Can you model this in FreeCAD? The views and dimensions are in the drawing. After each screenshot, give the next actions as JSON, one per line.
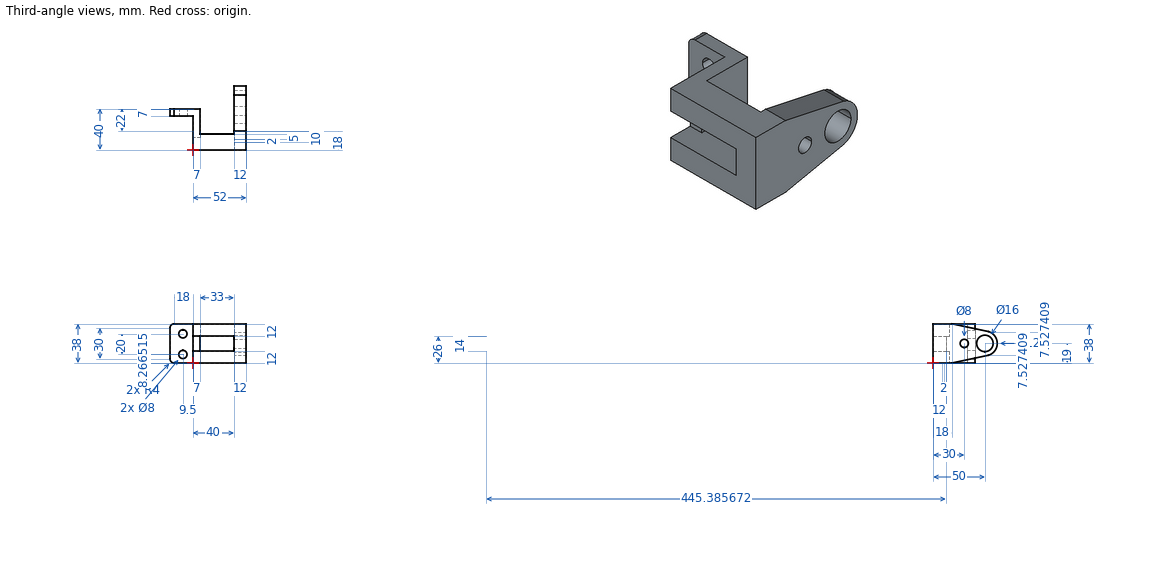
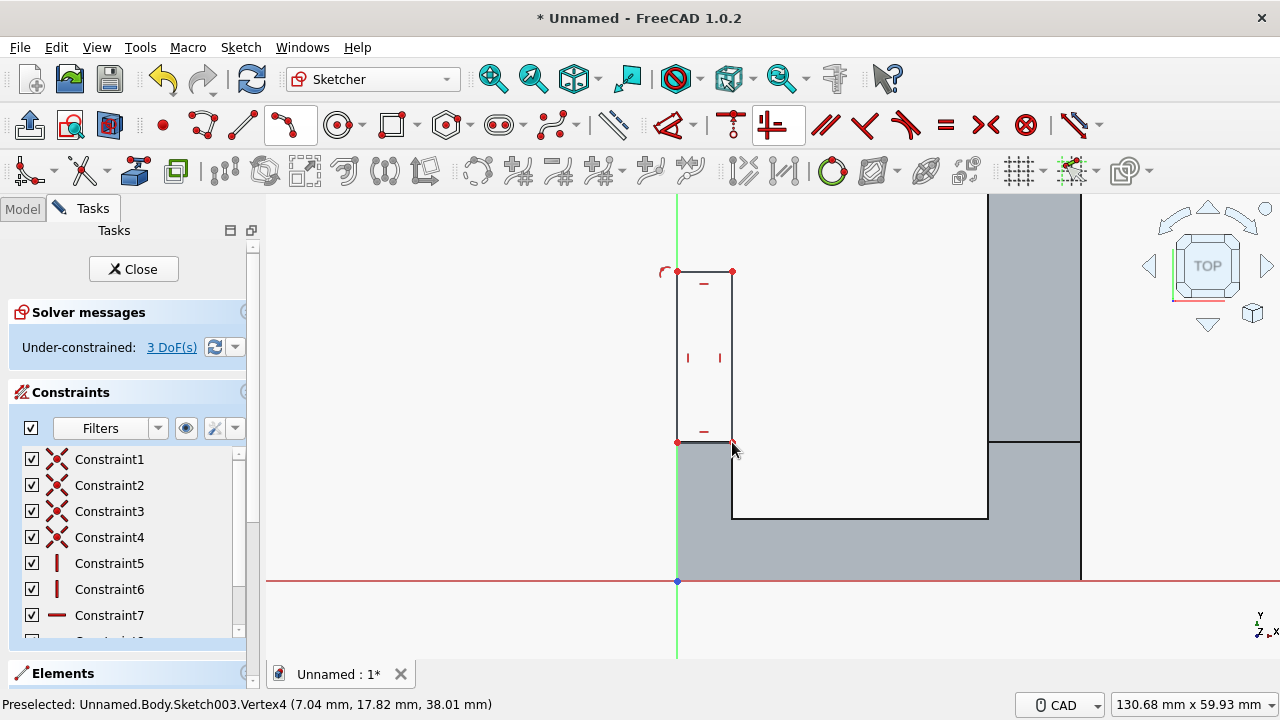
{"action": "left_click", "coordinate": [668, 126]}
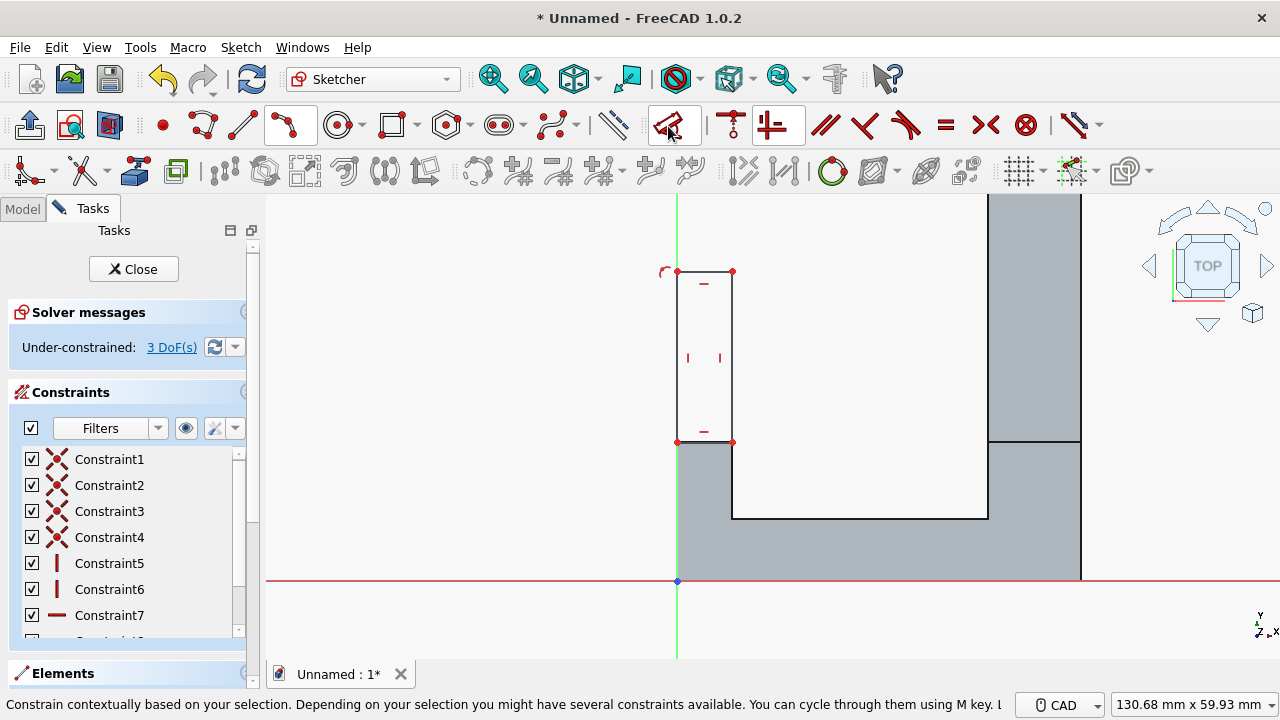
{"action": "left_click", "coordinate": [694, 443]}
{"action": "left_click", "coordinate": [705, 477]}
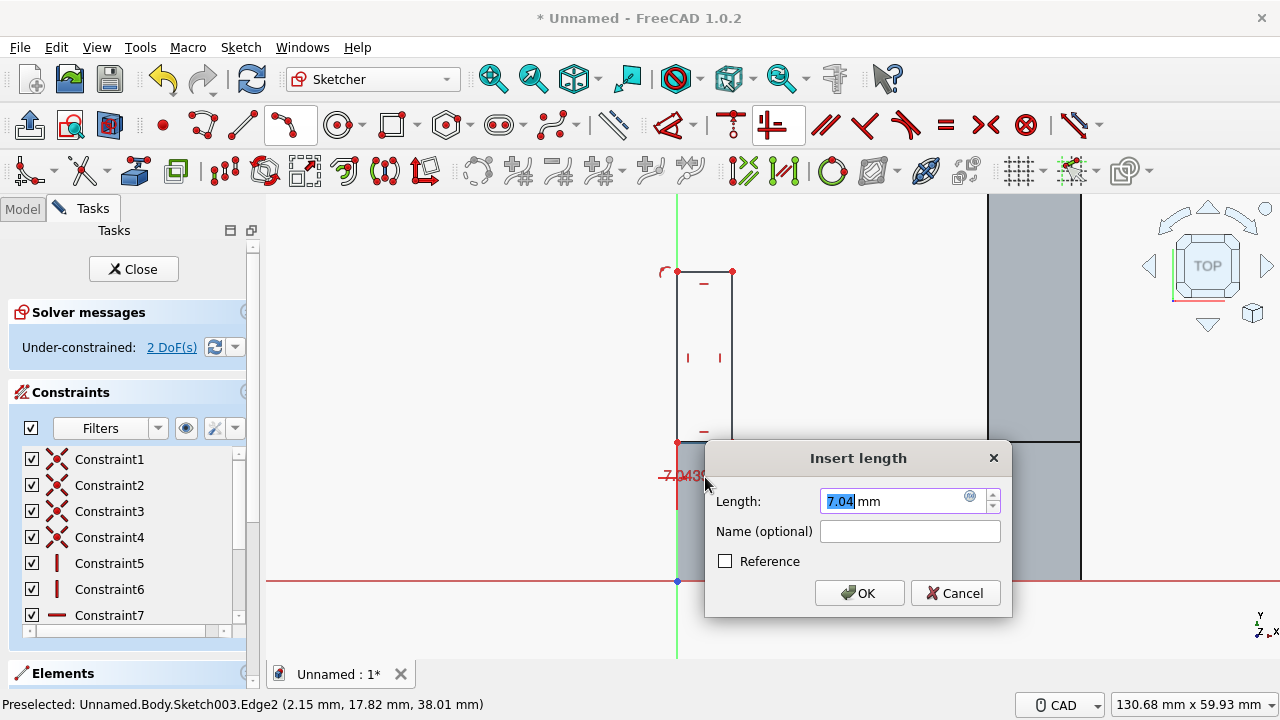
{"action": "type", "text": "7"}
{"action": "key", "text": "Return"}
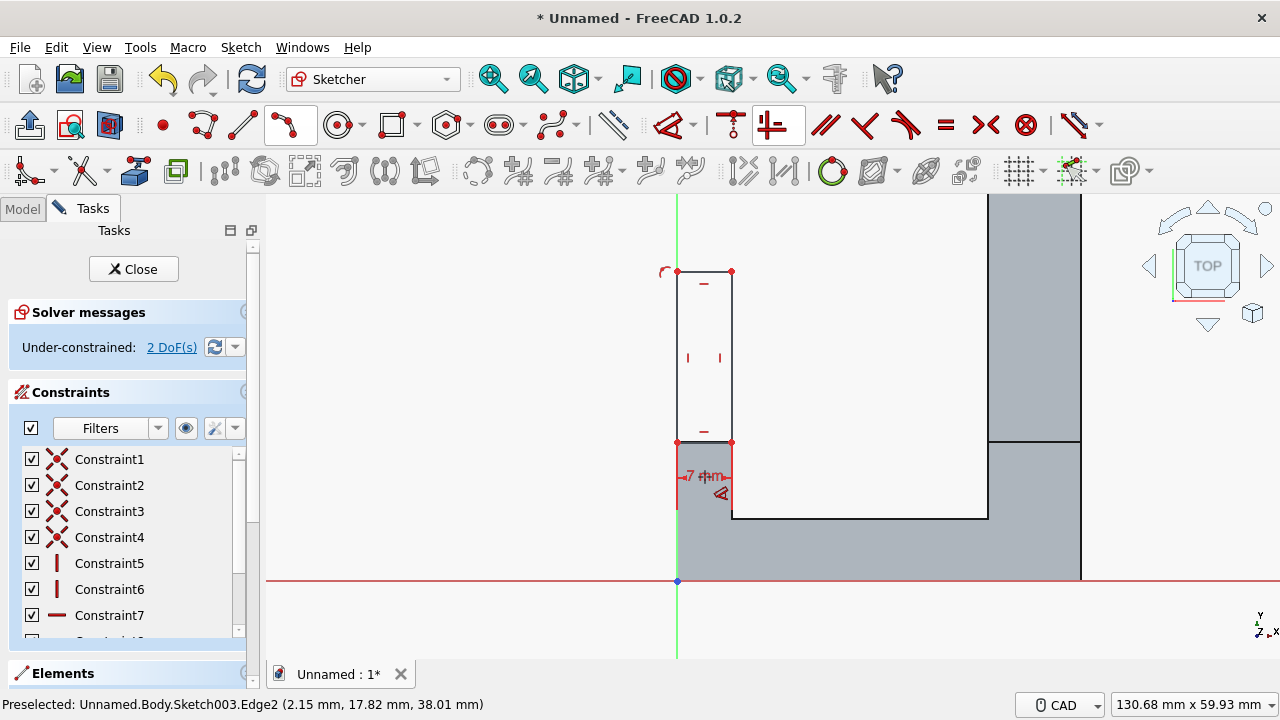
{"action": "left_click", "coordinate": [677, 323]}
{"action": "left_click", "coordinate": [643, 358]}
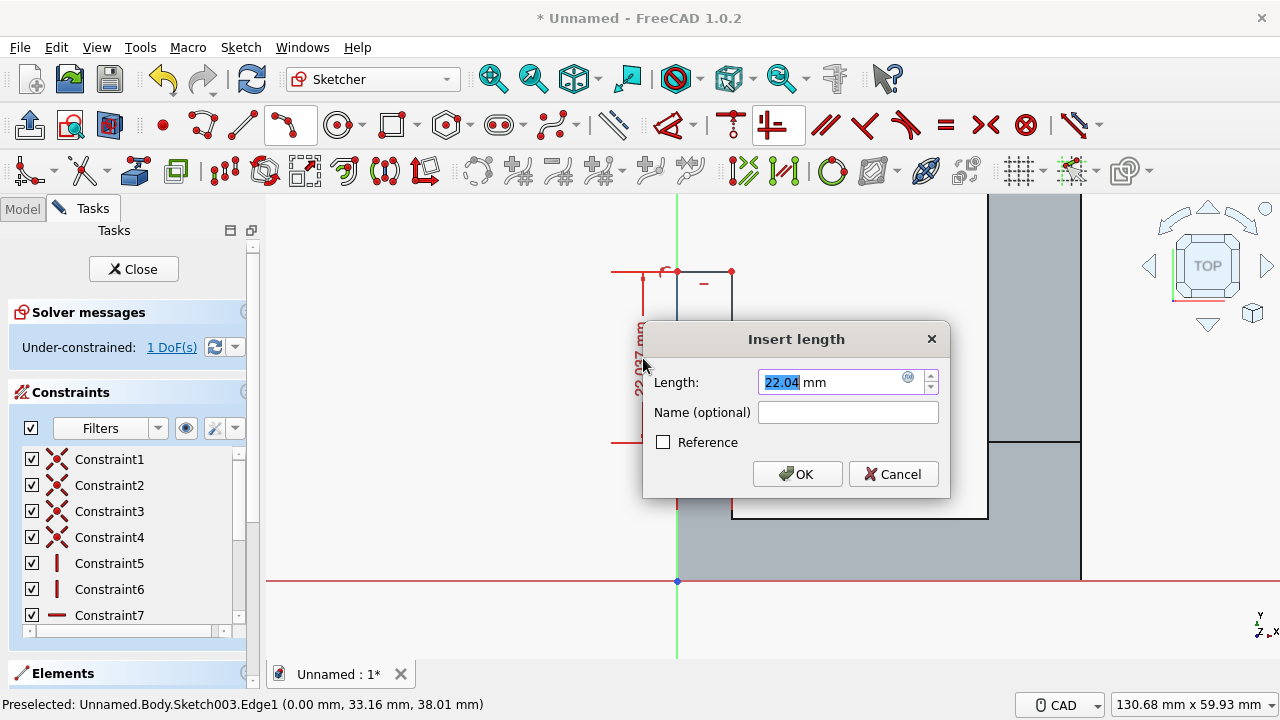
{"action": "type", "text": "22"}
{"action": "key", "text": "Return"}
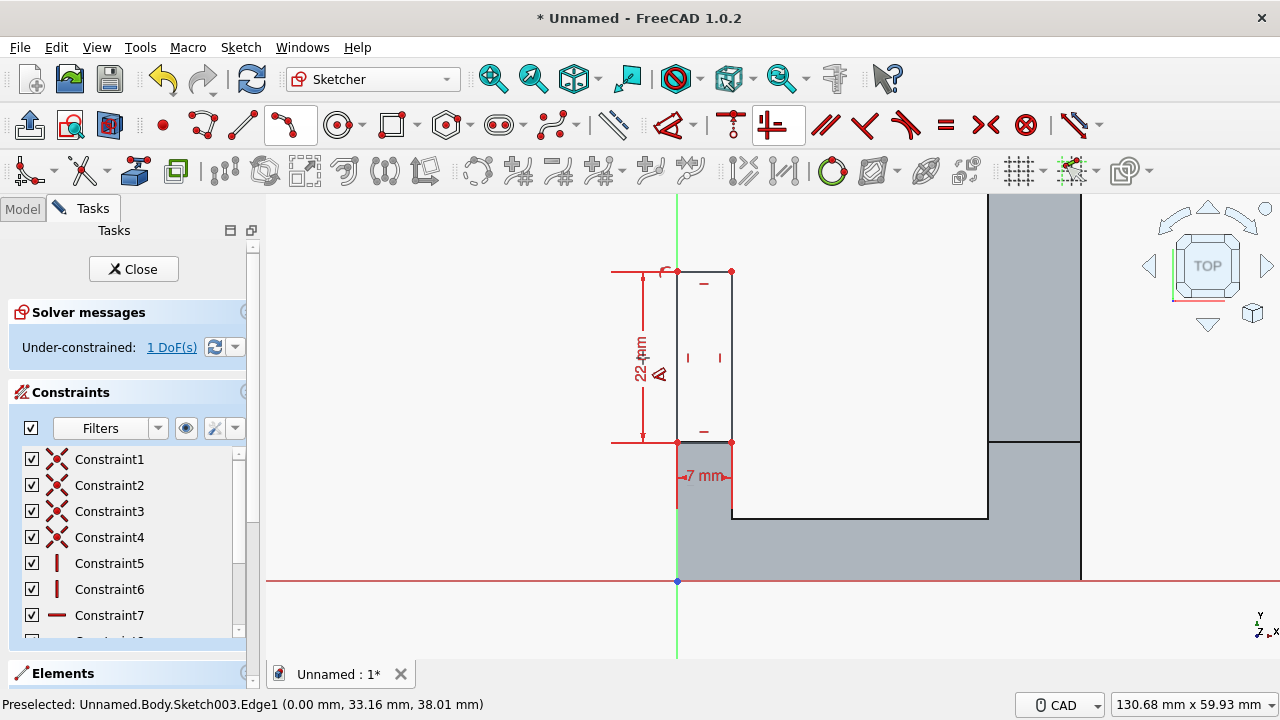
{"action": "left_click", "coordinate": [677, 272]}
{"action": "left_click", "coordinate": [643, 427]}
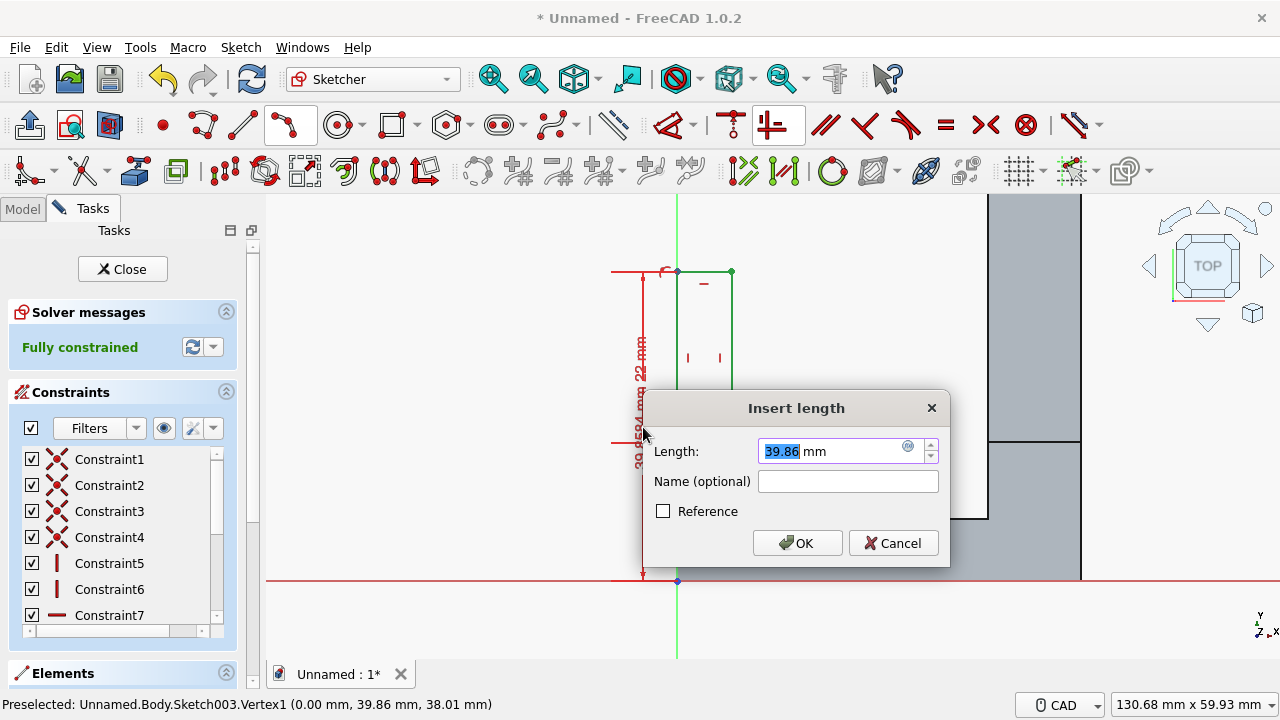
{"action": "type", "text": "40"}
{"action": "key", "text": "Return"}
{"action": "key", "text": "Escape"}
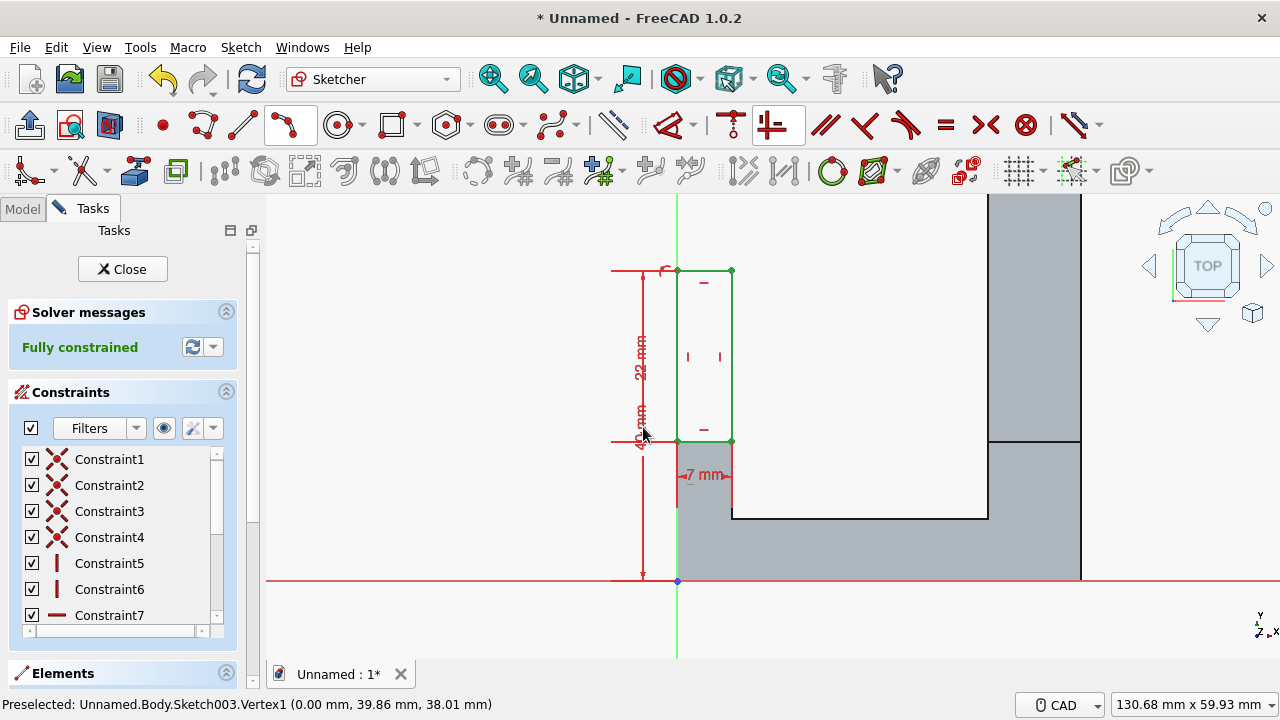
{"action": "left_click", "coordinate": [123, 269]}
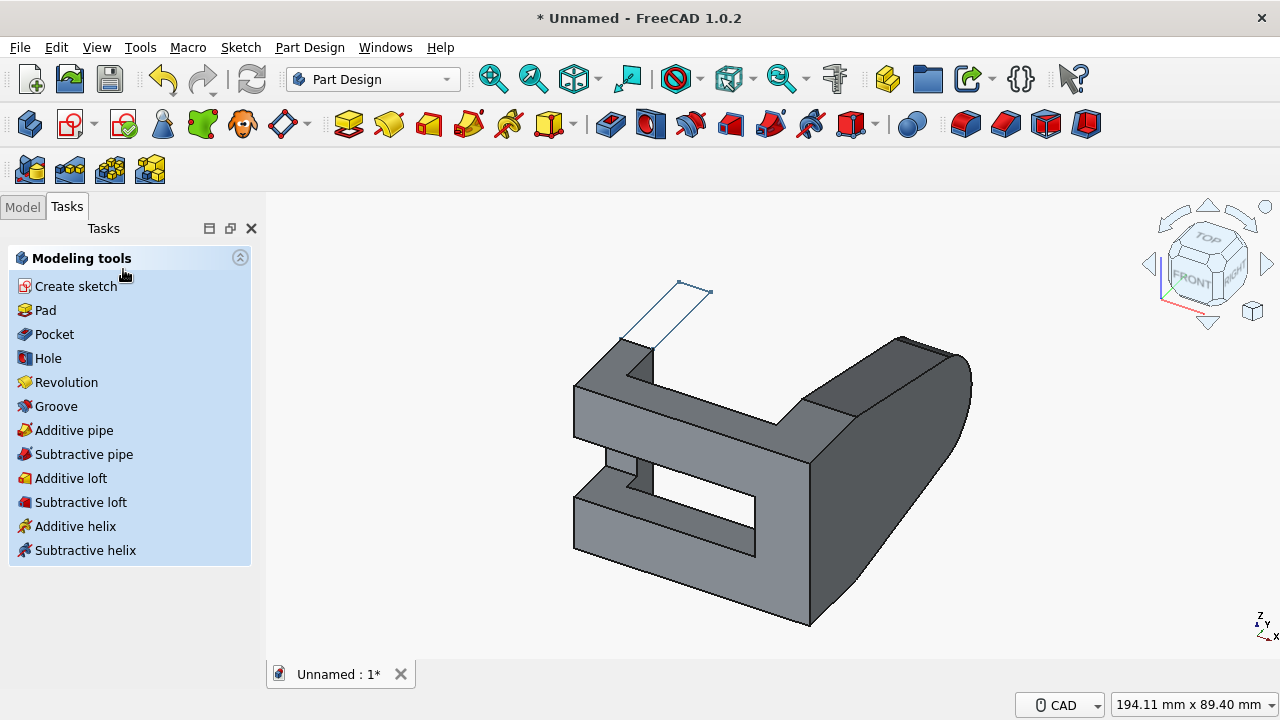
{"action": "left_click", "coordinate": [350, 124]}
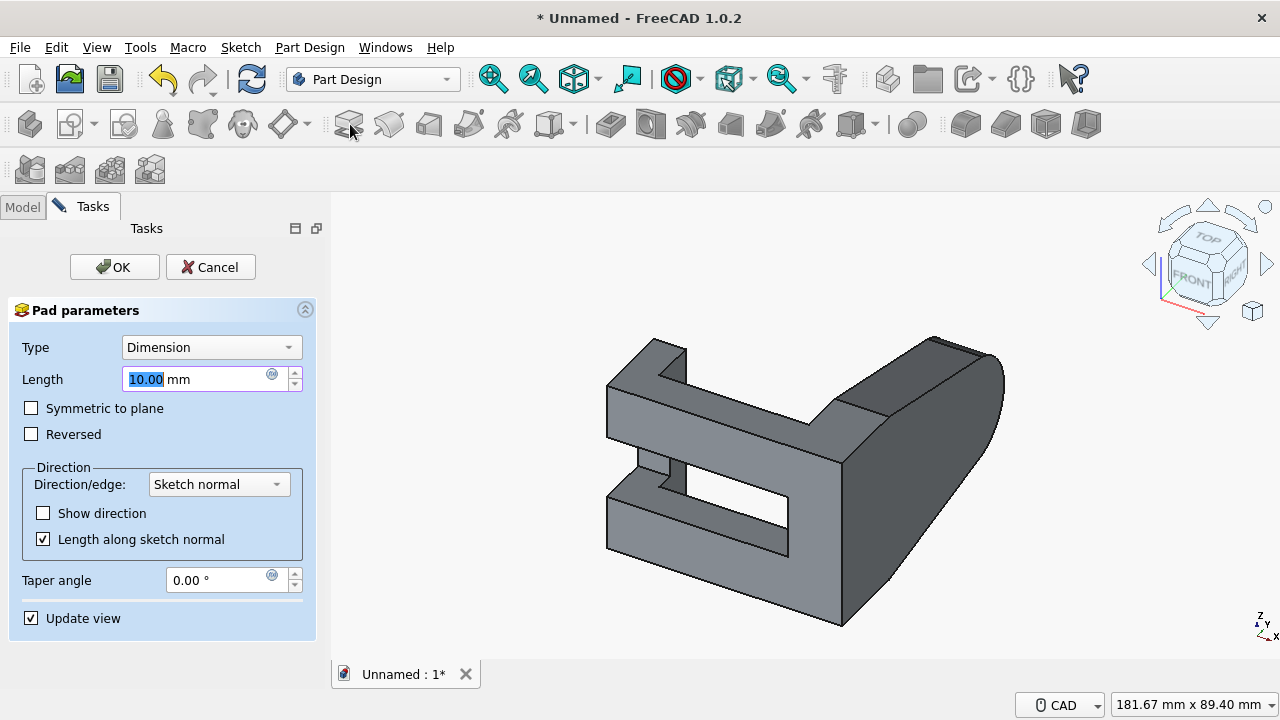
{"action": "type", "text": "38"}
{"action": "key", "text": "Tab"}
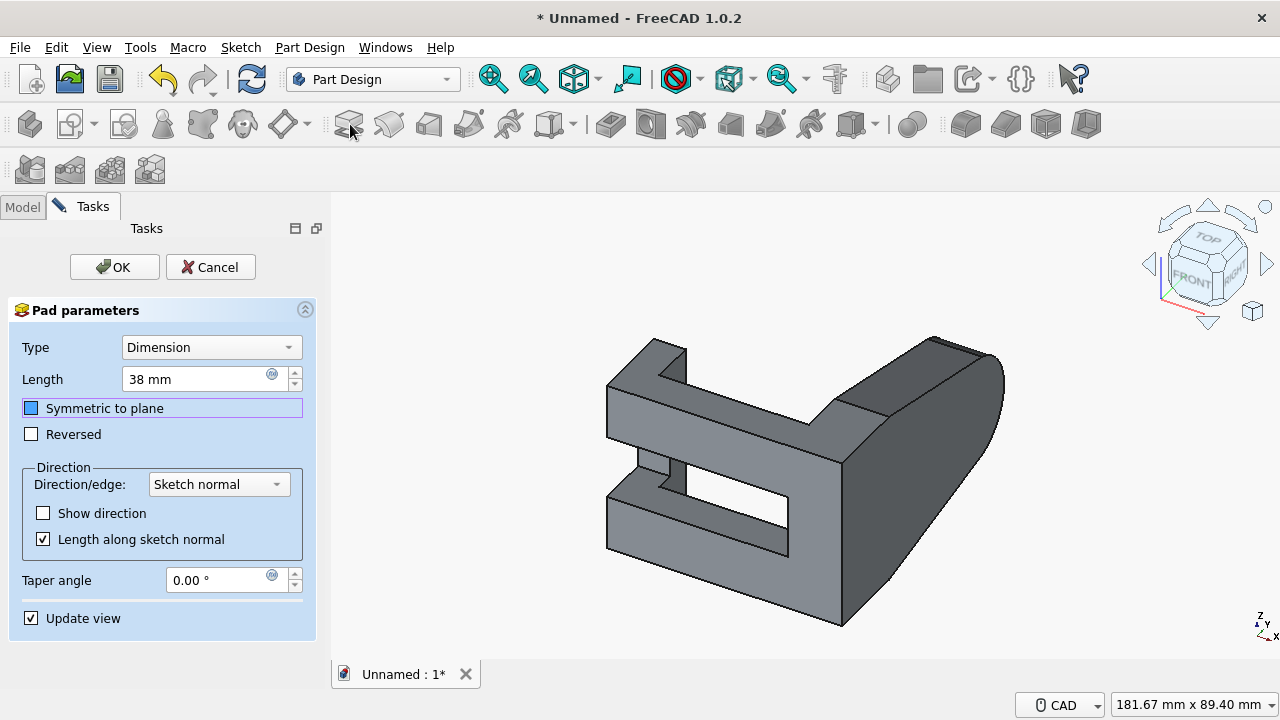
{"action": "left_click", "coordinate": [30, 434]}